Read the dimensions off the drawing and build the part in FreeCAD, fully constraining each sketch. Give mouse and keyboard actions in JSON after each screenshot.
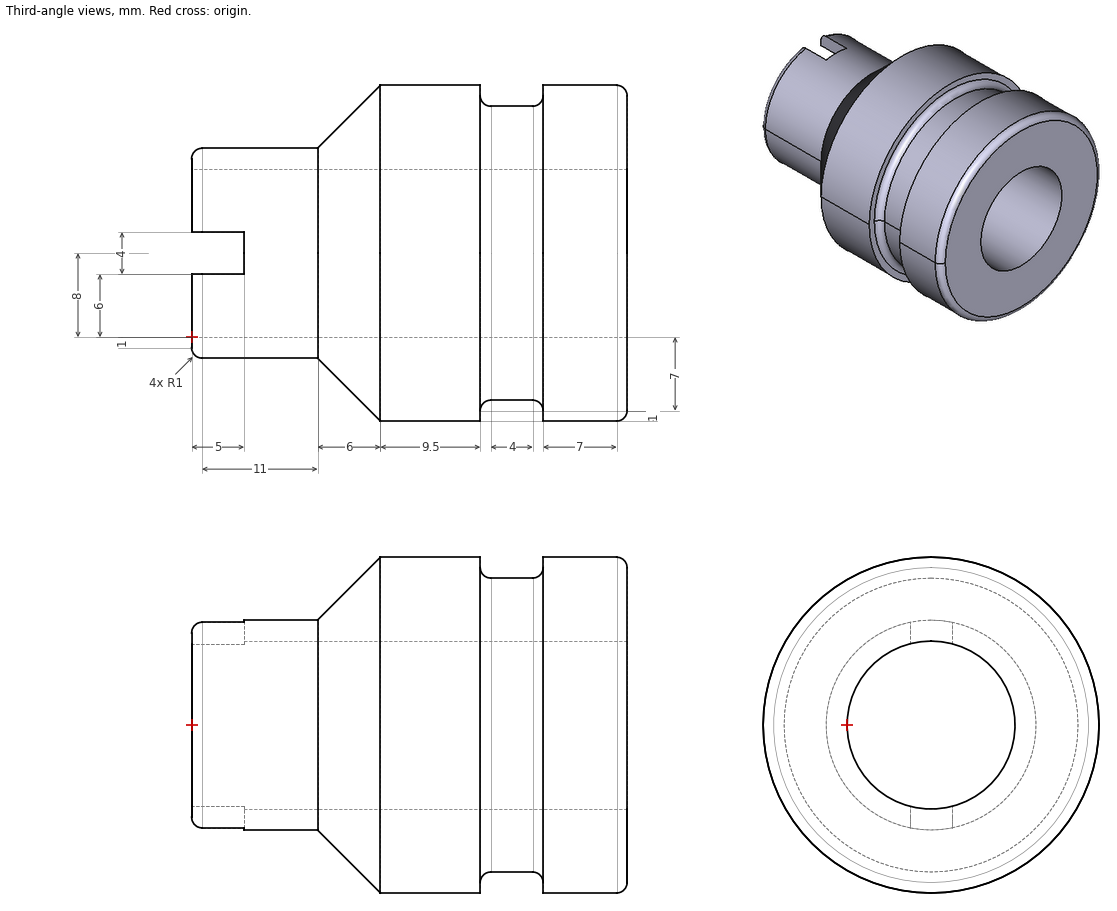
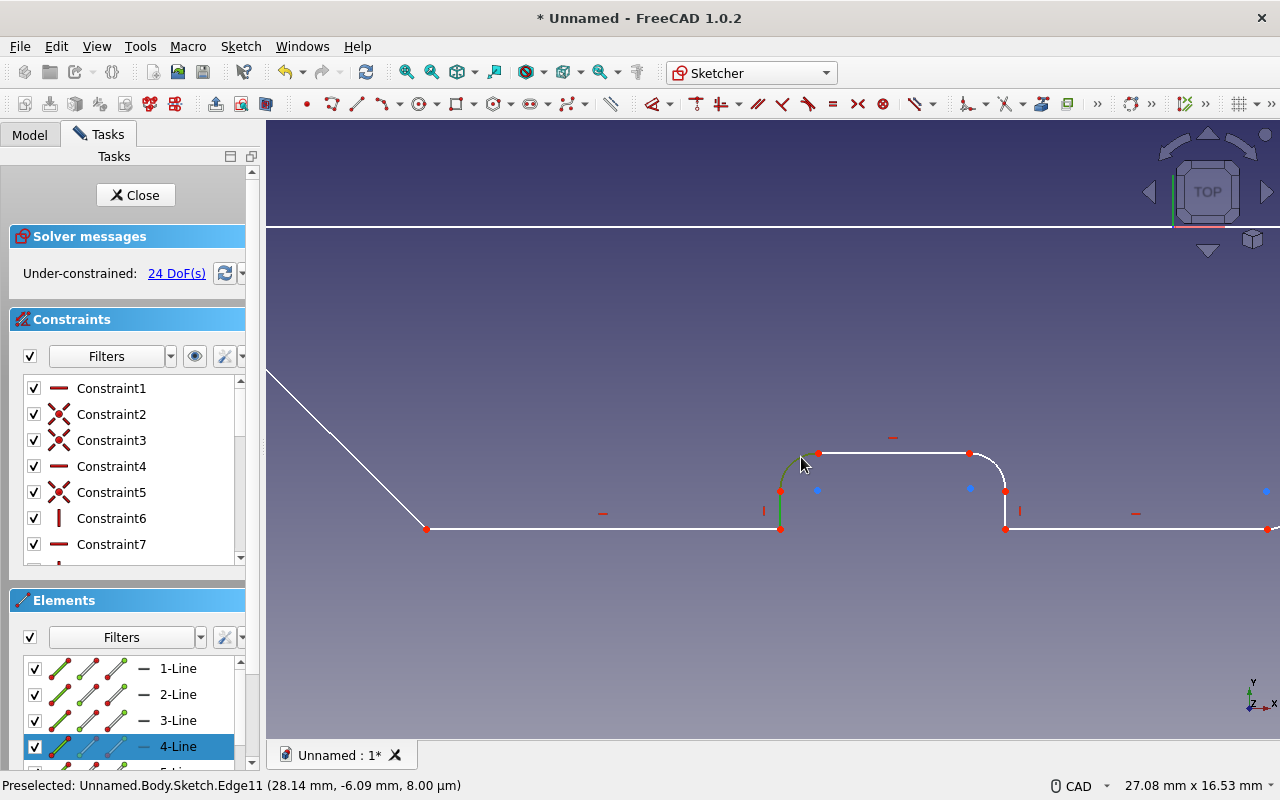
{"action": "key", "text": "t"}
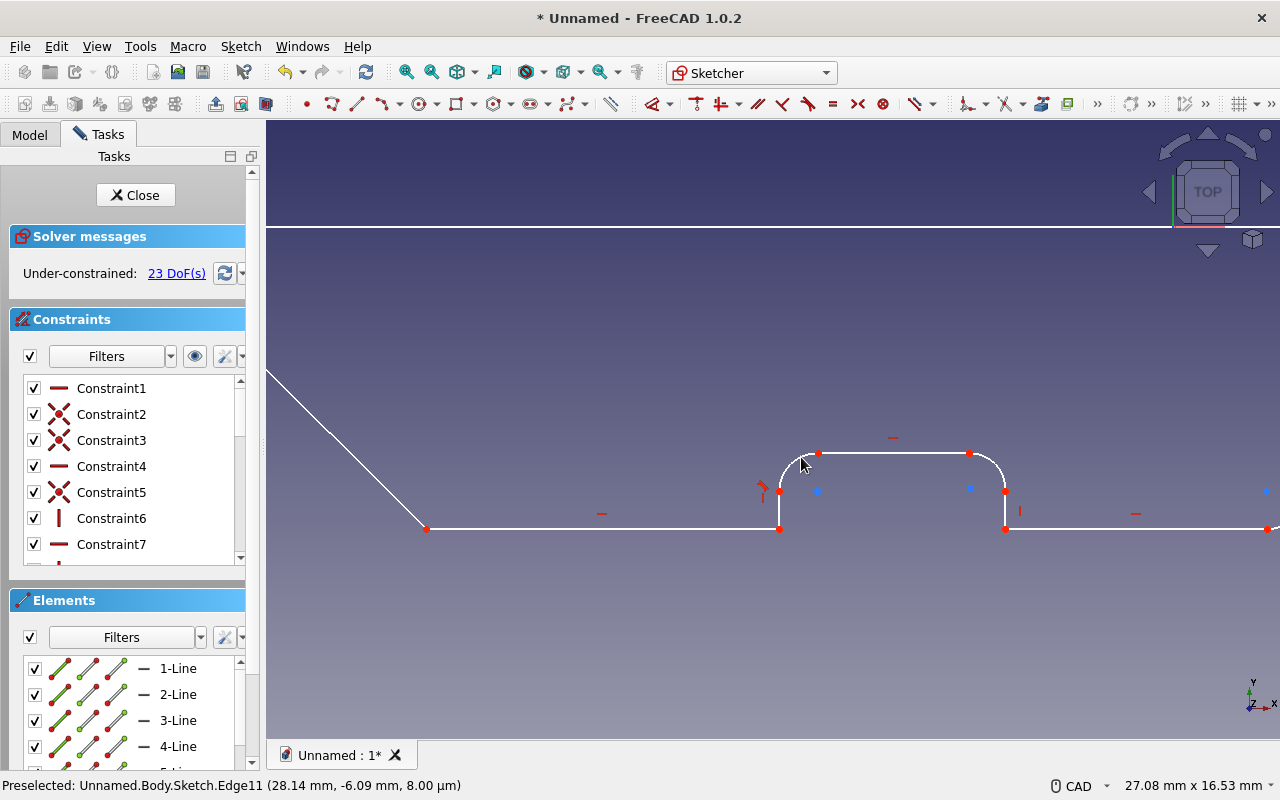
{"action": "left_click", "coordinate": [864, 453]}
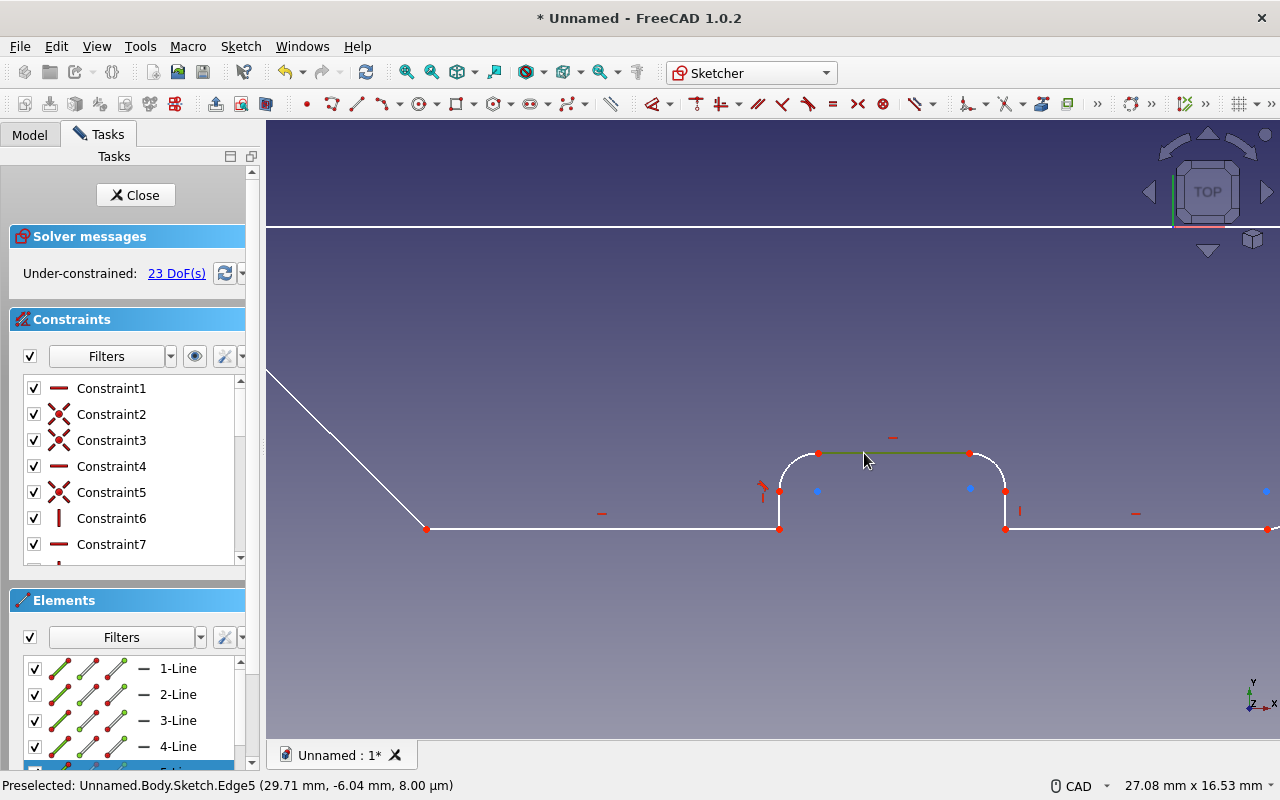
{"action": "left_click", "coordinate": [801, 457]}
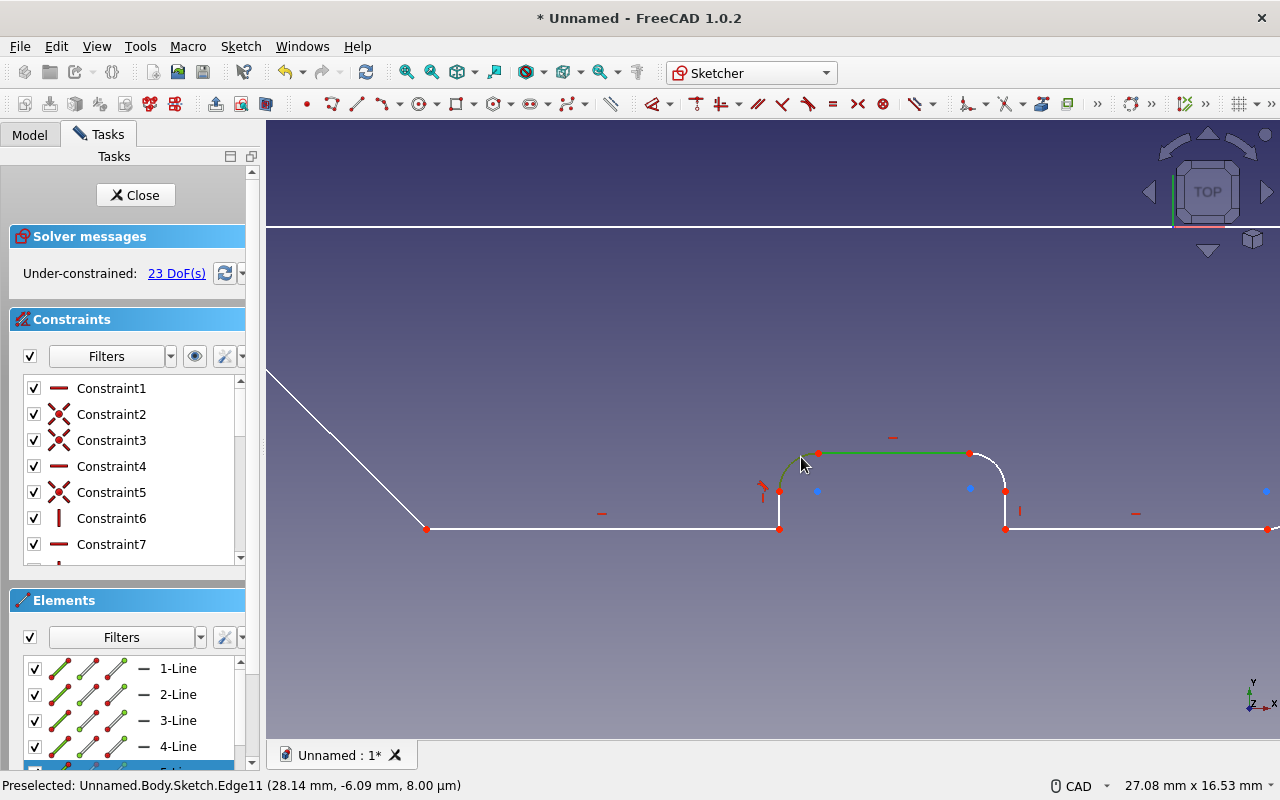
{"action": "key", "text": "t"}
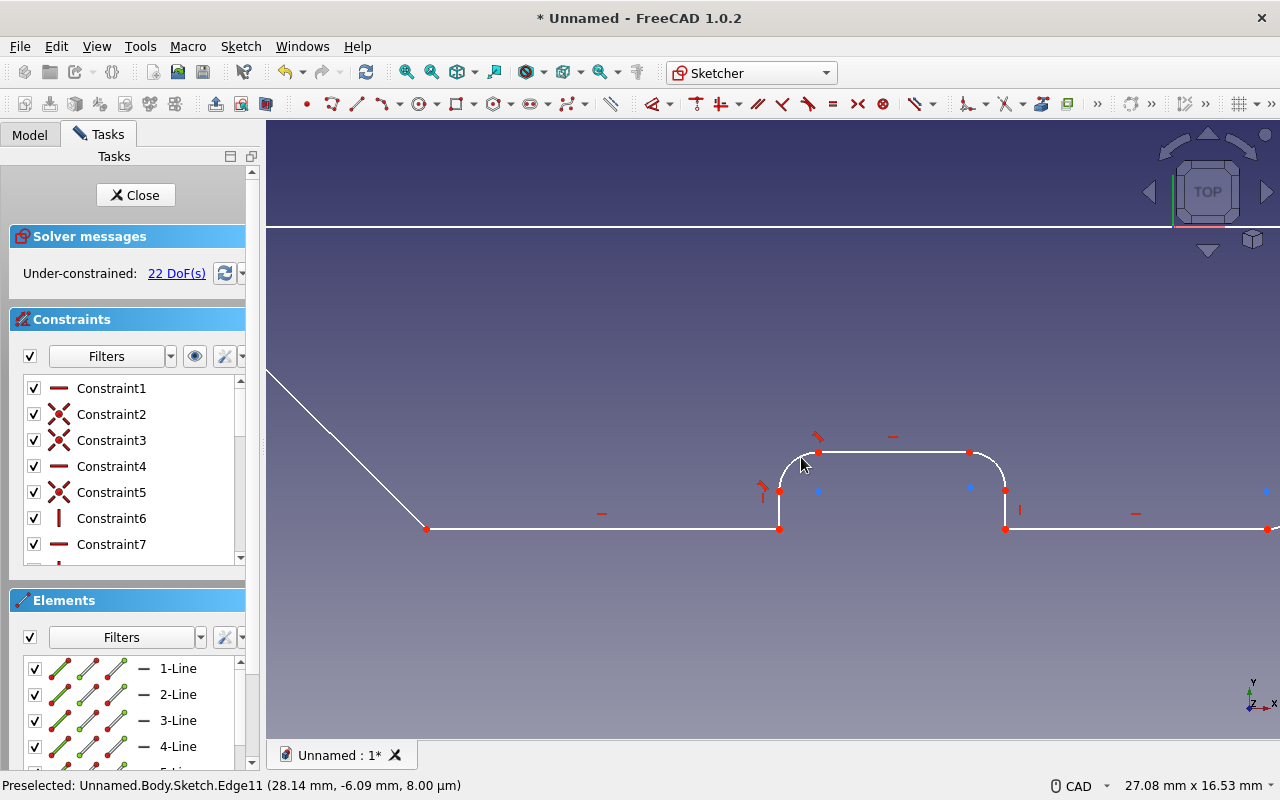
{"action": "left_click", "coordinate": [864, 452]}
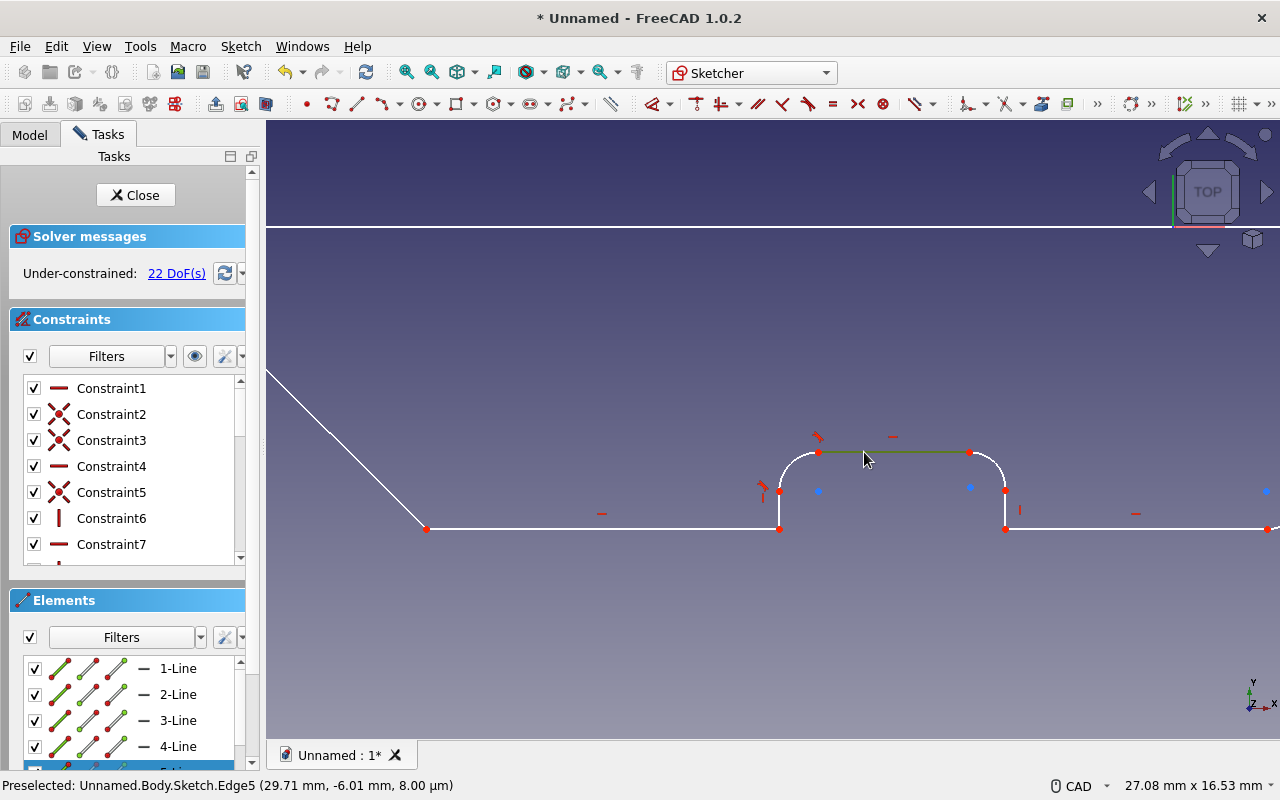
{"action": "left_click", "coordinate": [1002, 473]}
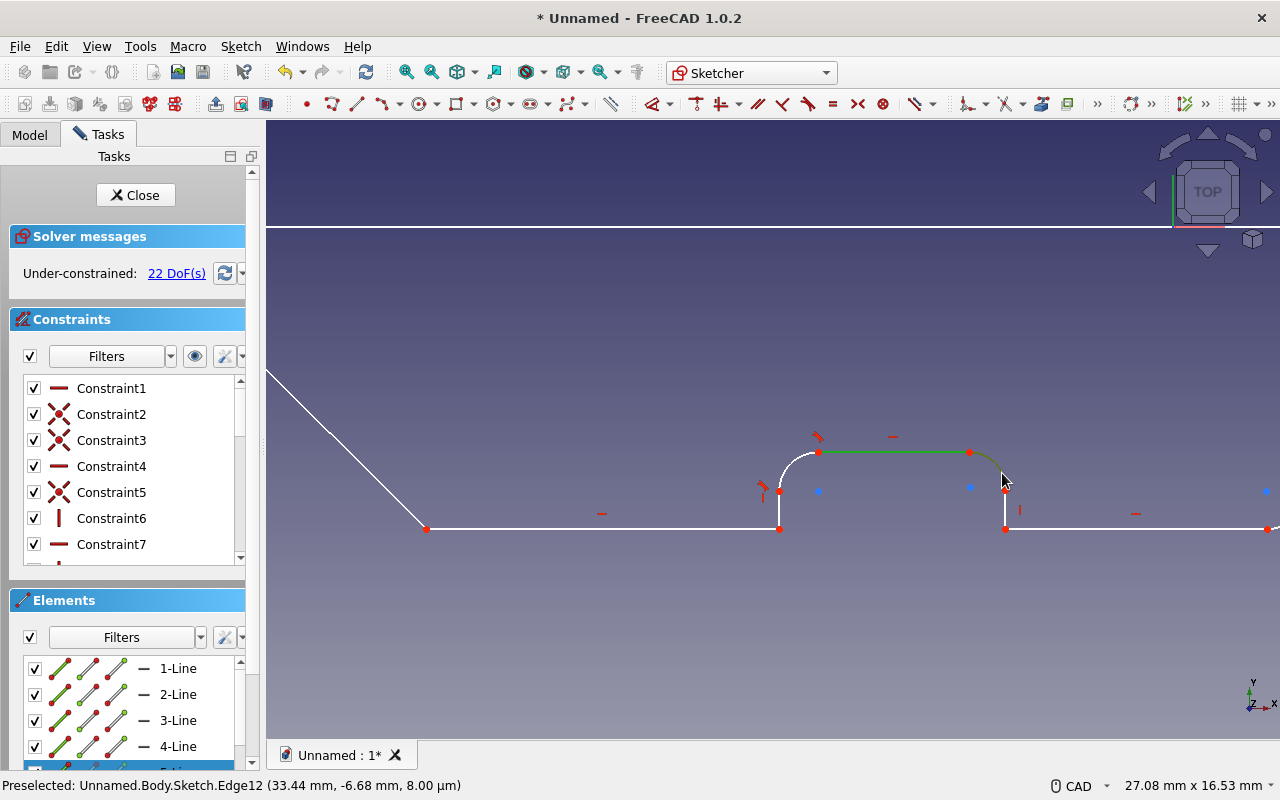
{"action": "key", "text": "t"}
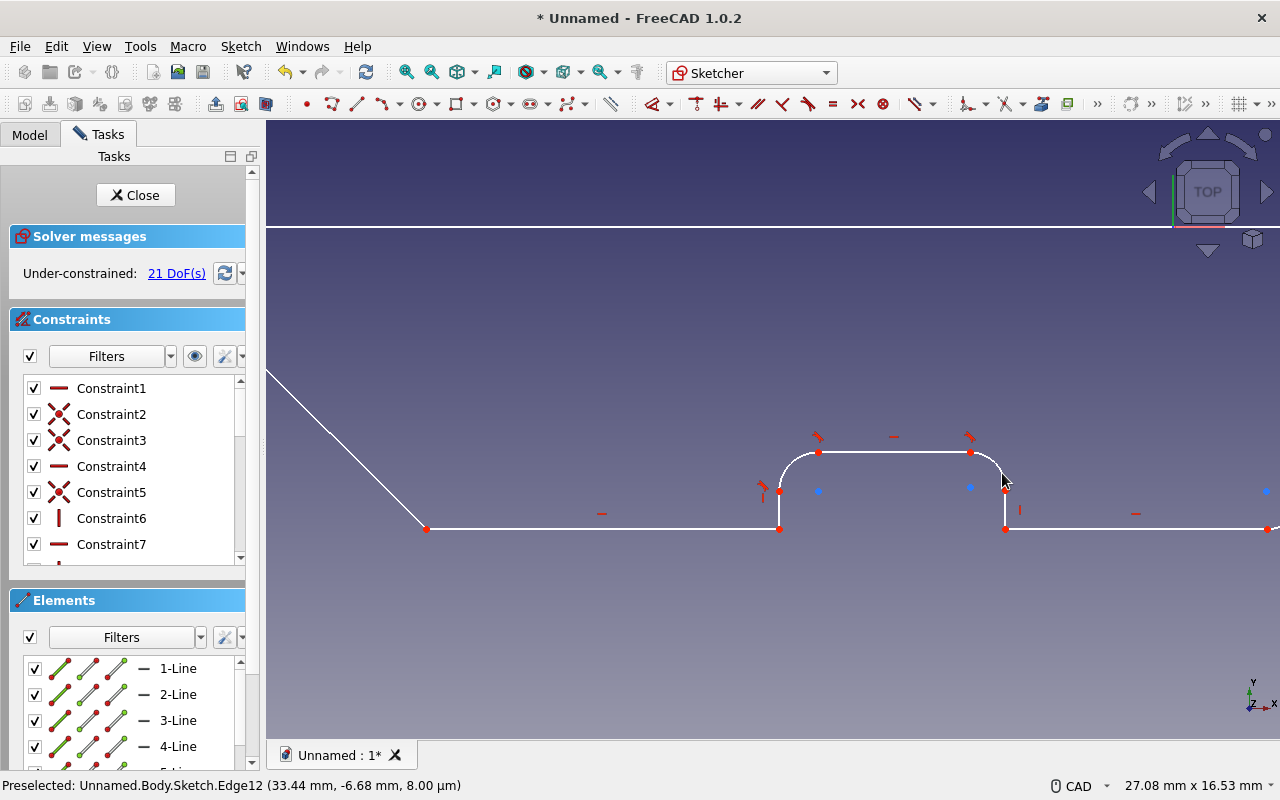
{"action": "left_click", "coordinate": [1005, 502]}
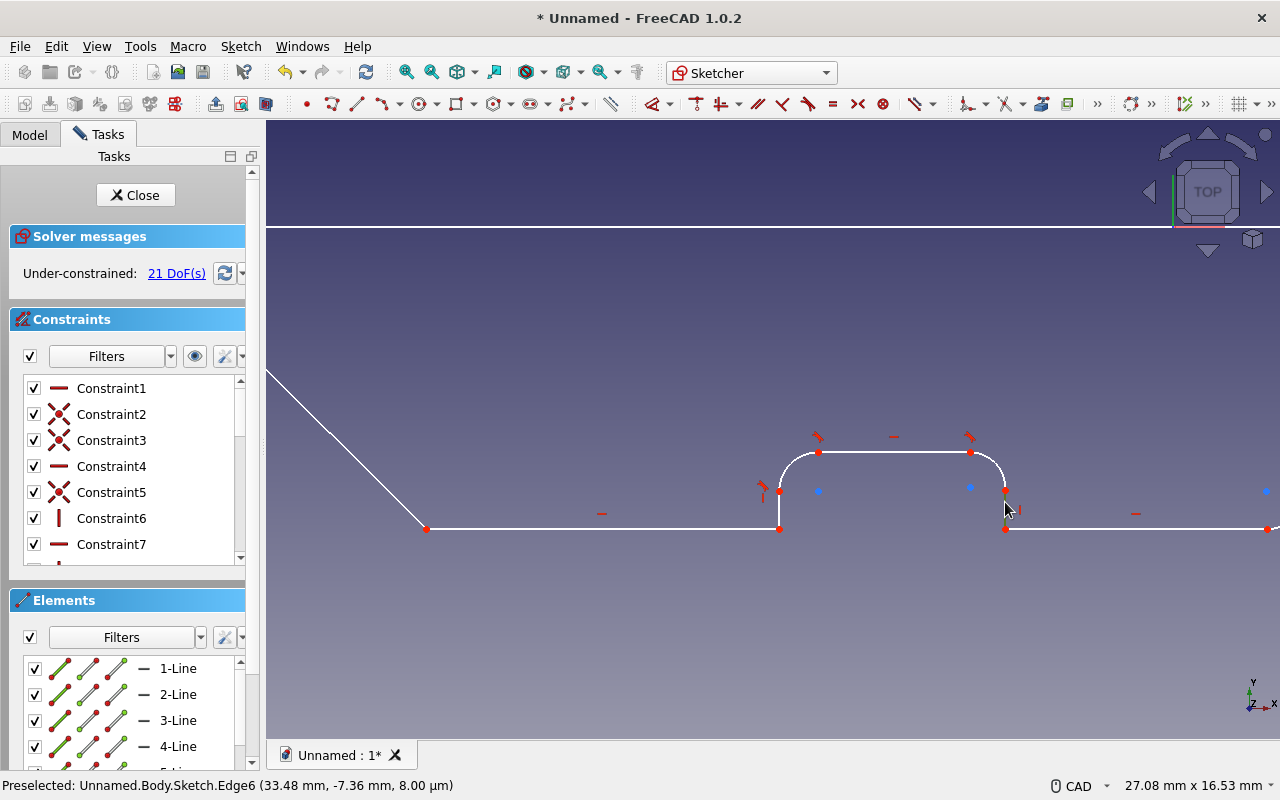
{"action": "left_click", "coordinate": [1002, 473]}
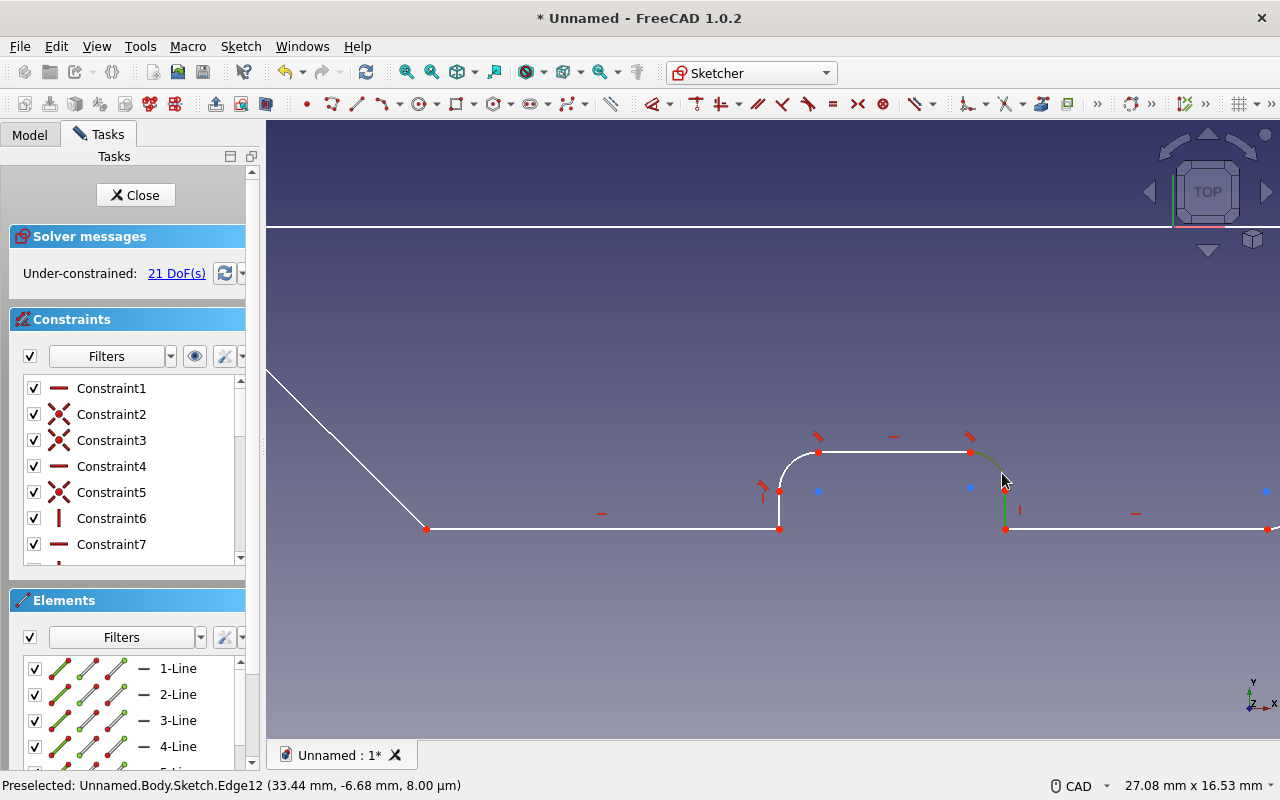
{"action": "left_click", "coordinate": [808, 104]}